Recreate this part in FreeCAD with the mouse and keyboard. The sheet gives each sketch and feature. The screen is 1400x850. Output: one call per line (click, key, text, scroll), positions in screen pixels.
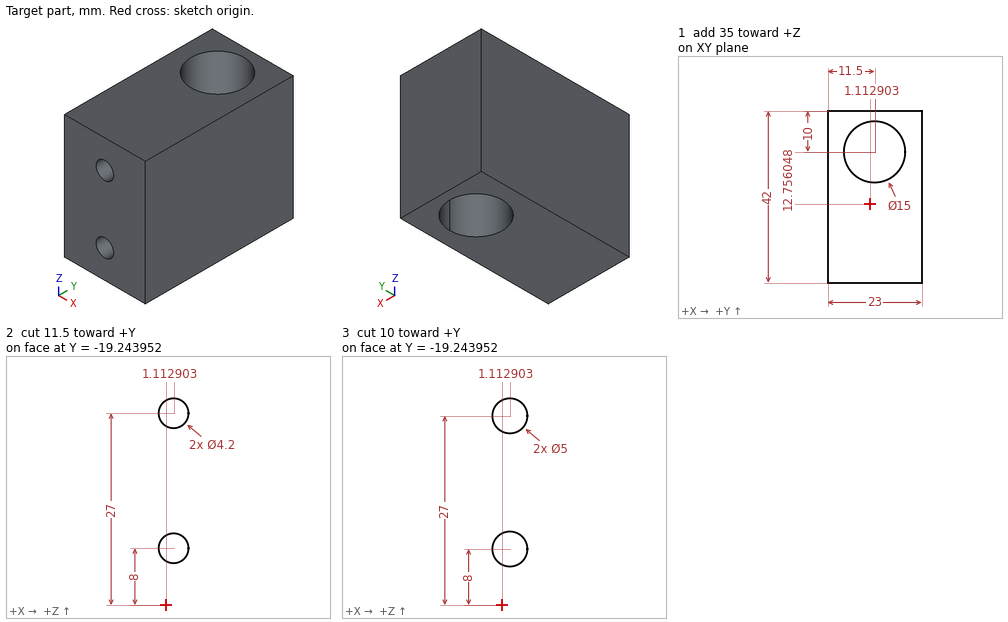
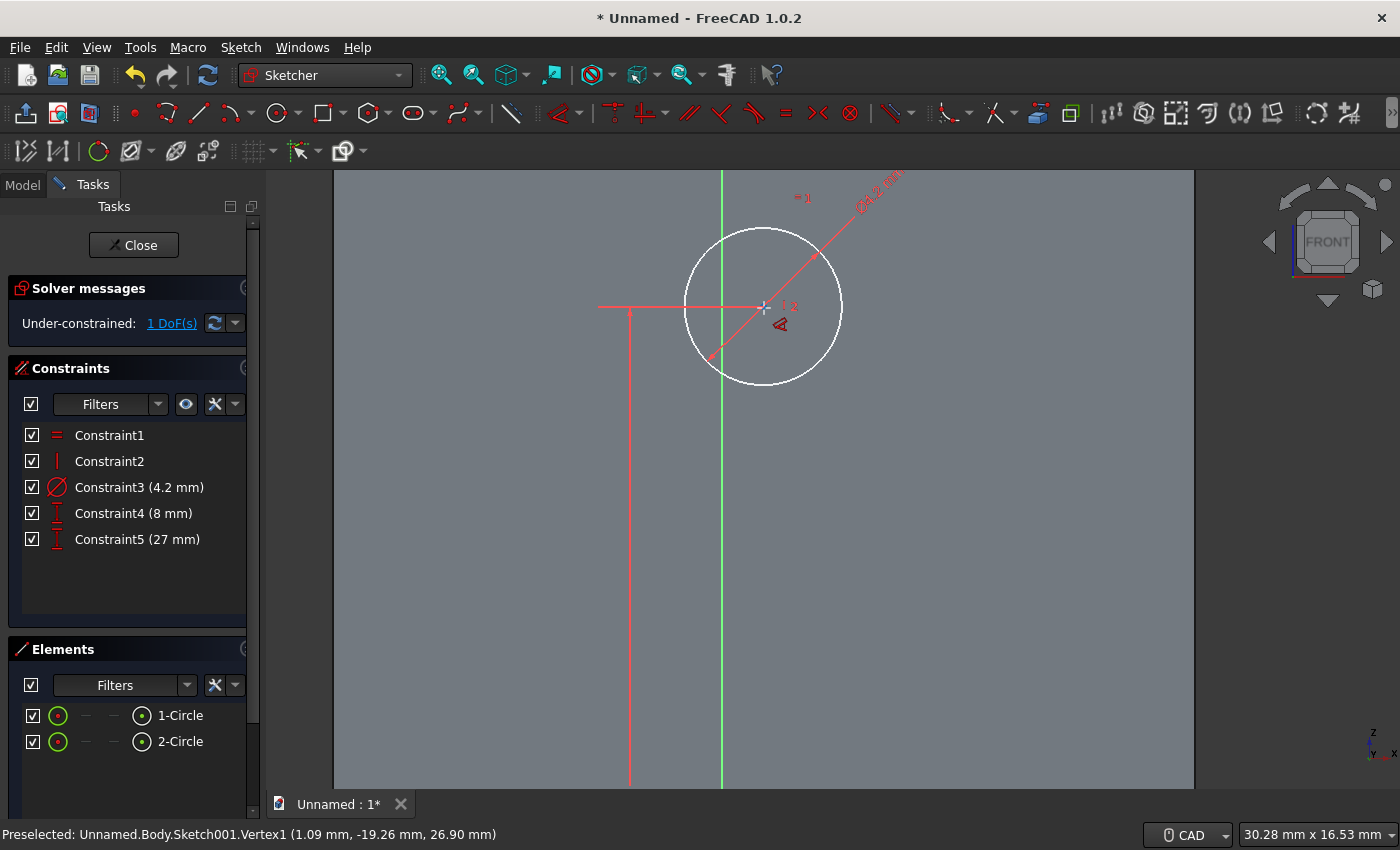
click(763, 307)
click(743, 273)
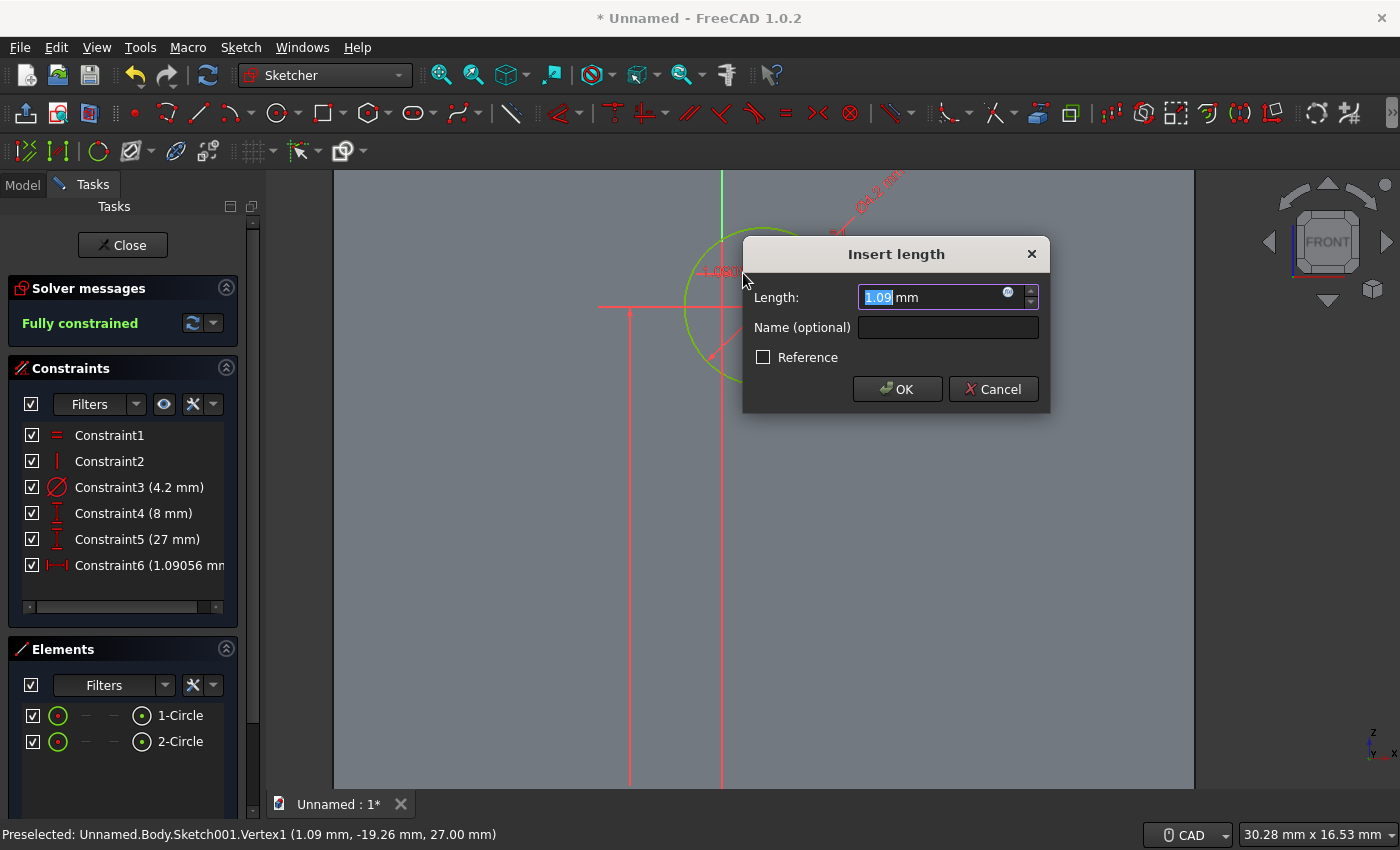
text(1.112903)
key(Return)
key(Escape)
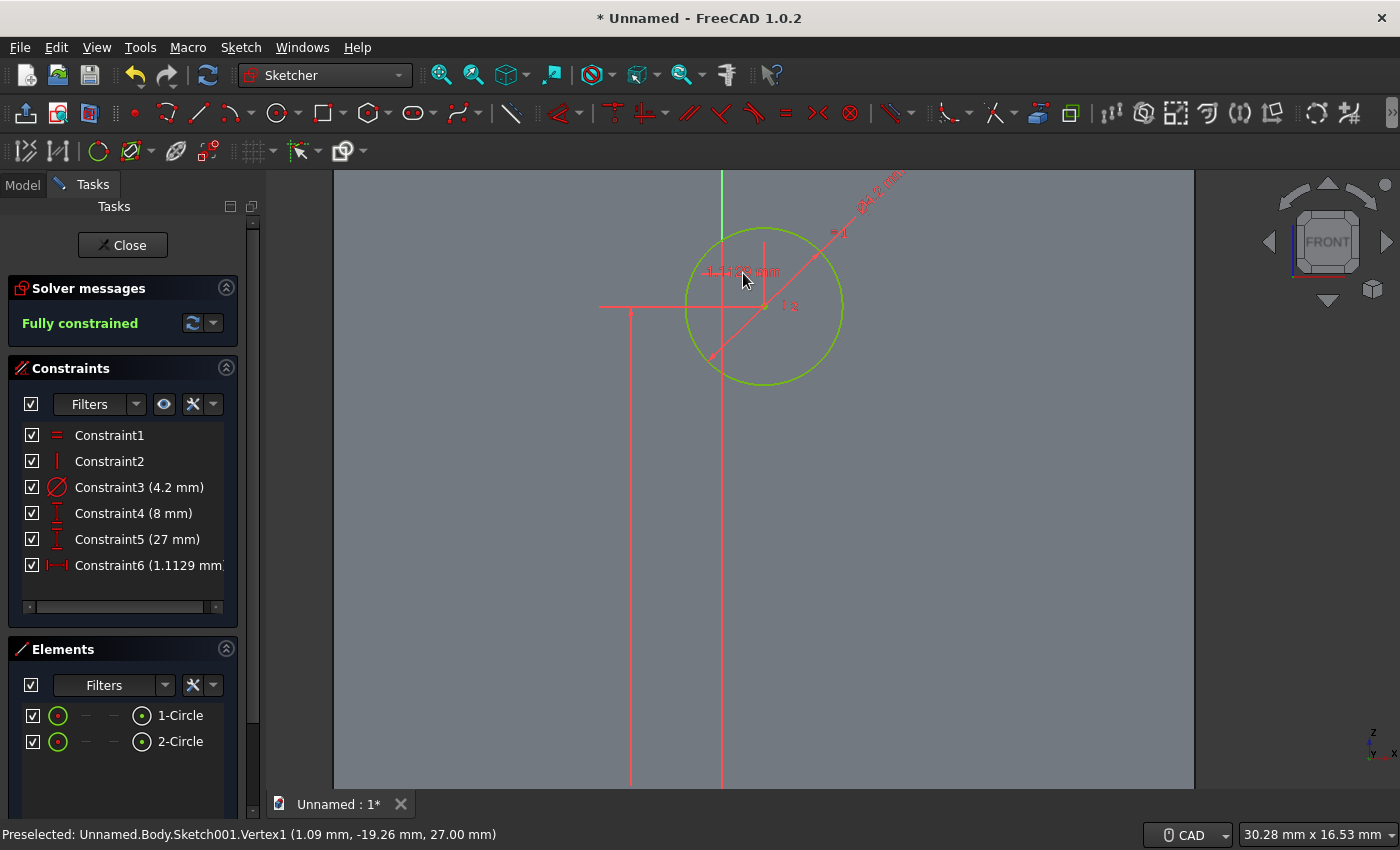
click(123, 245)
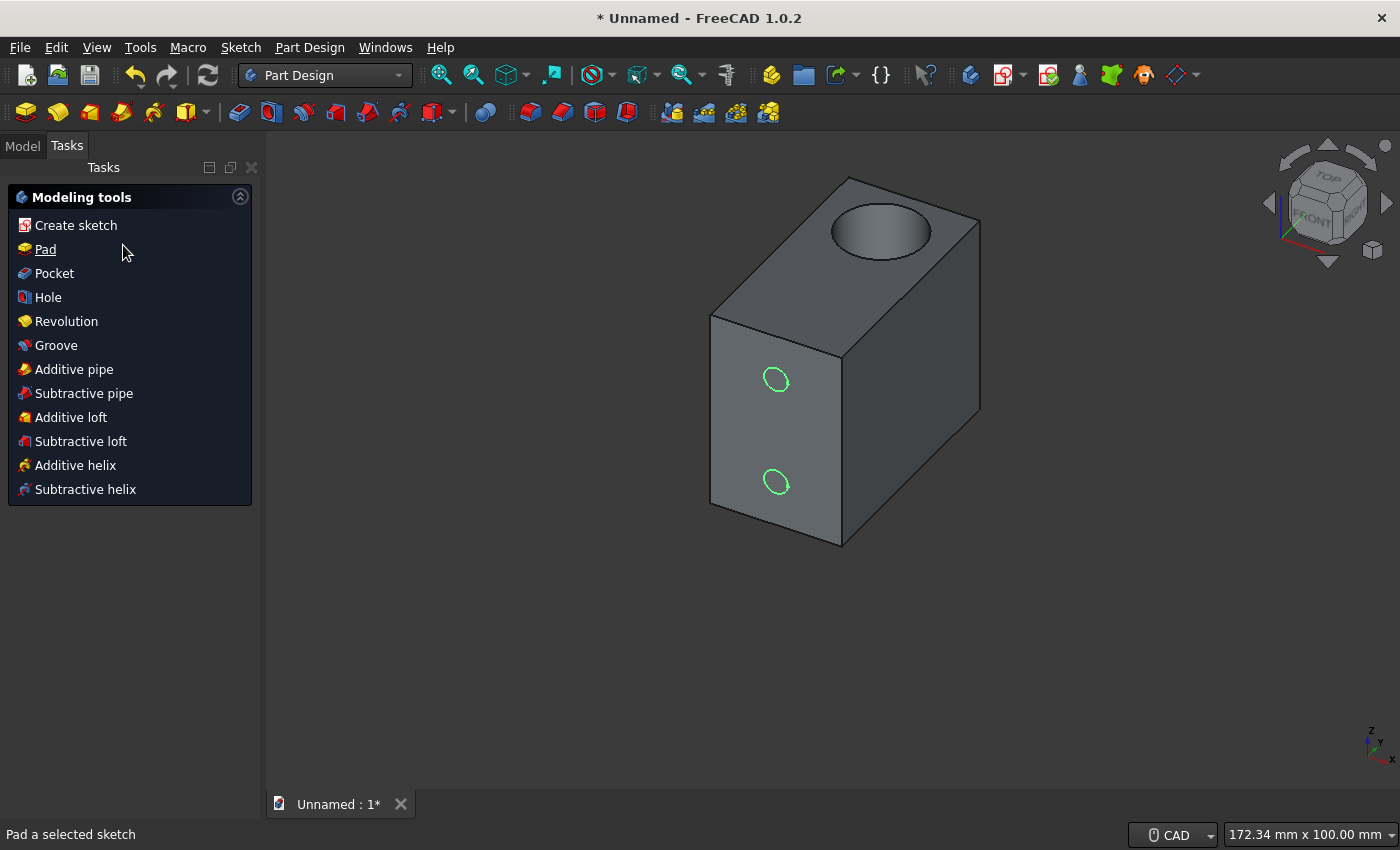
click(240, 112)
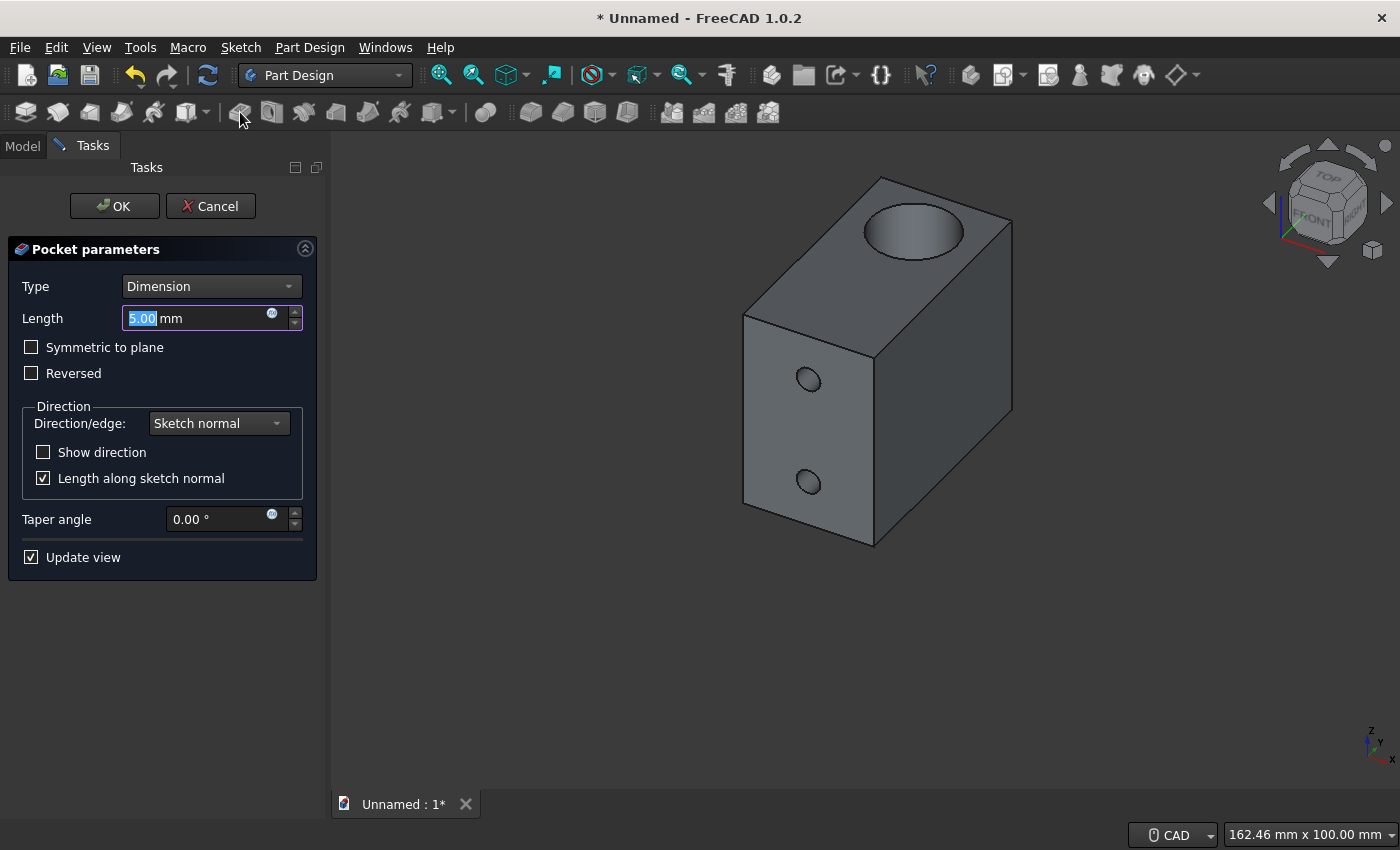
text(11.5)
key(Tab)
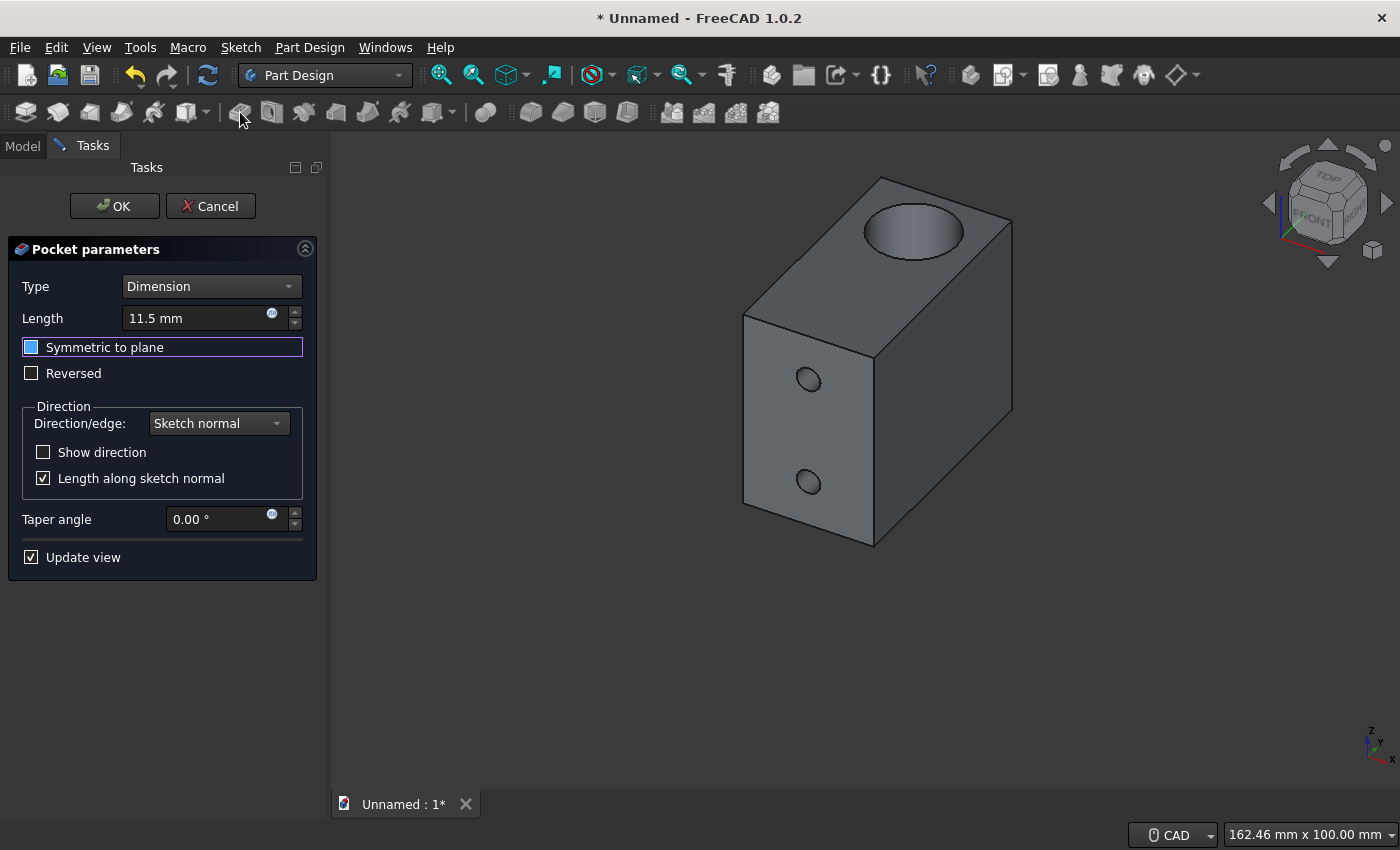
click(115, 206)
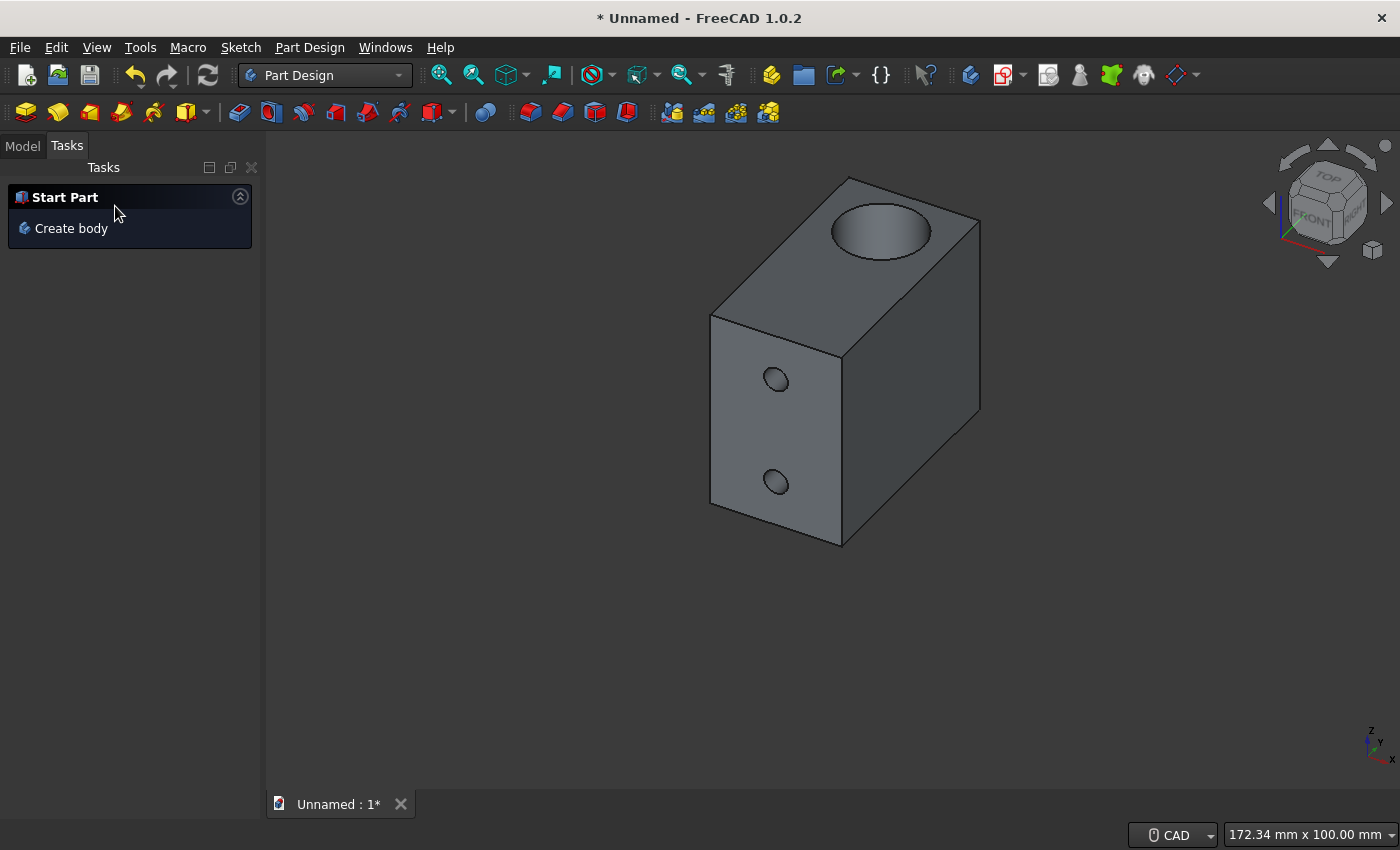
click(795, 436)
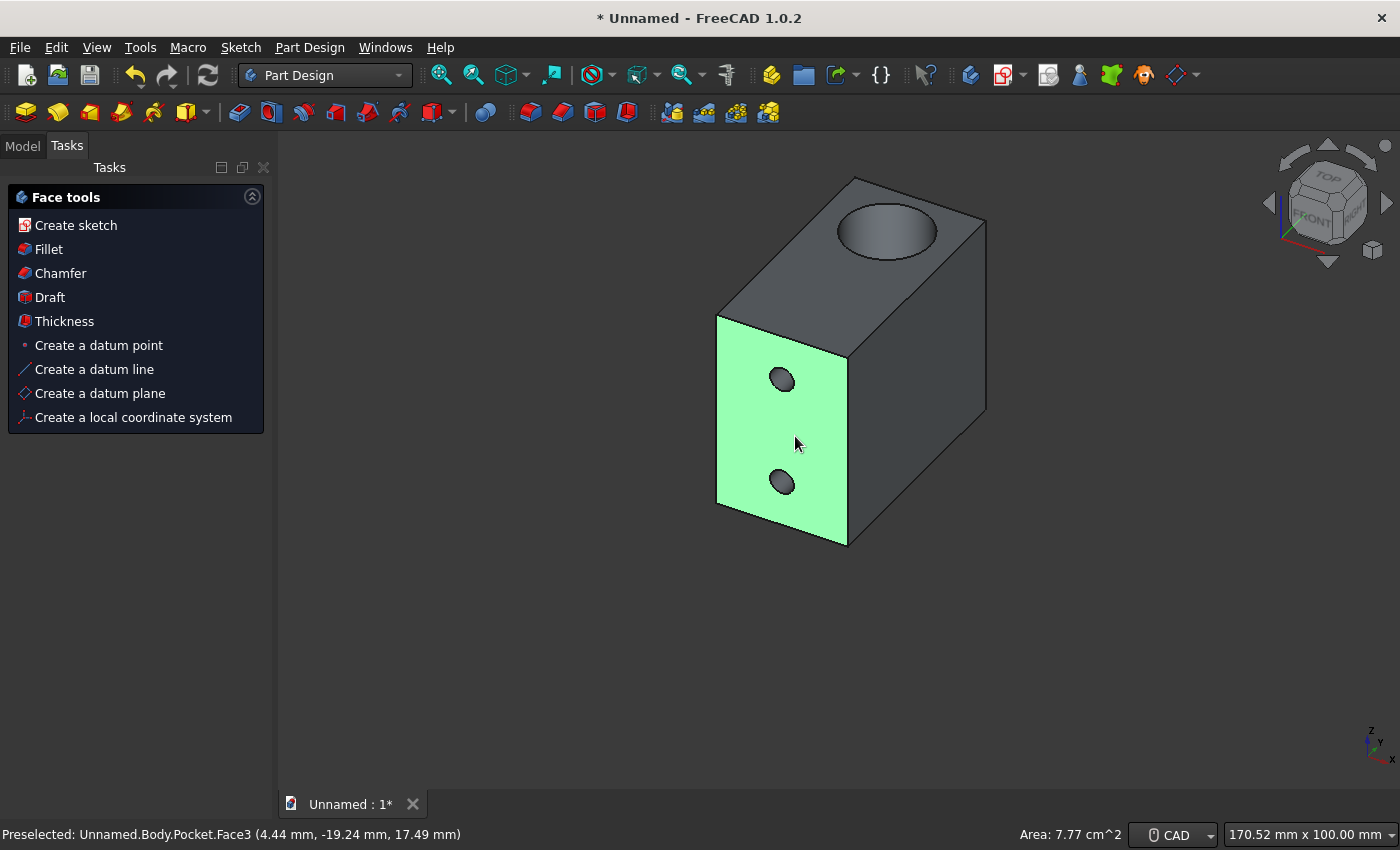
click(1004, 76)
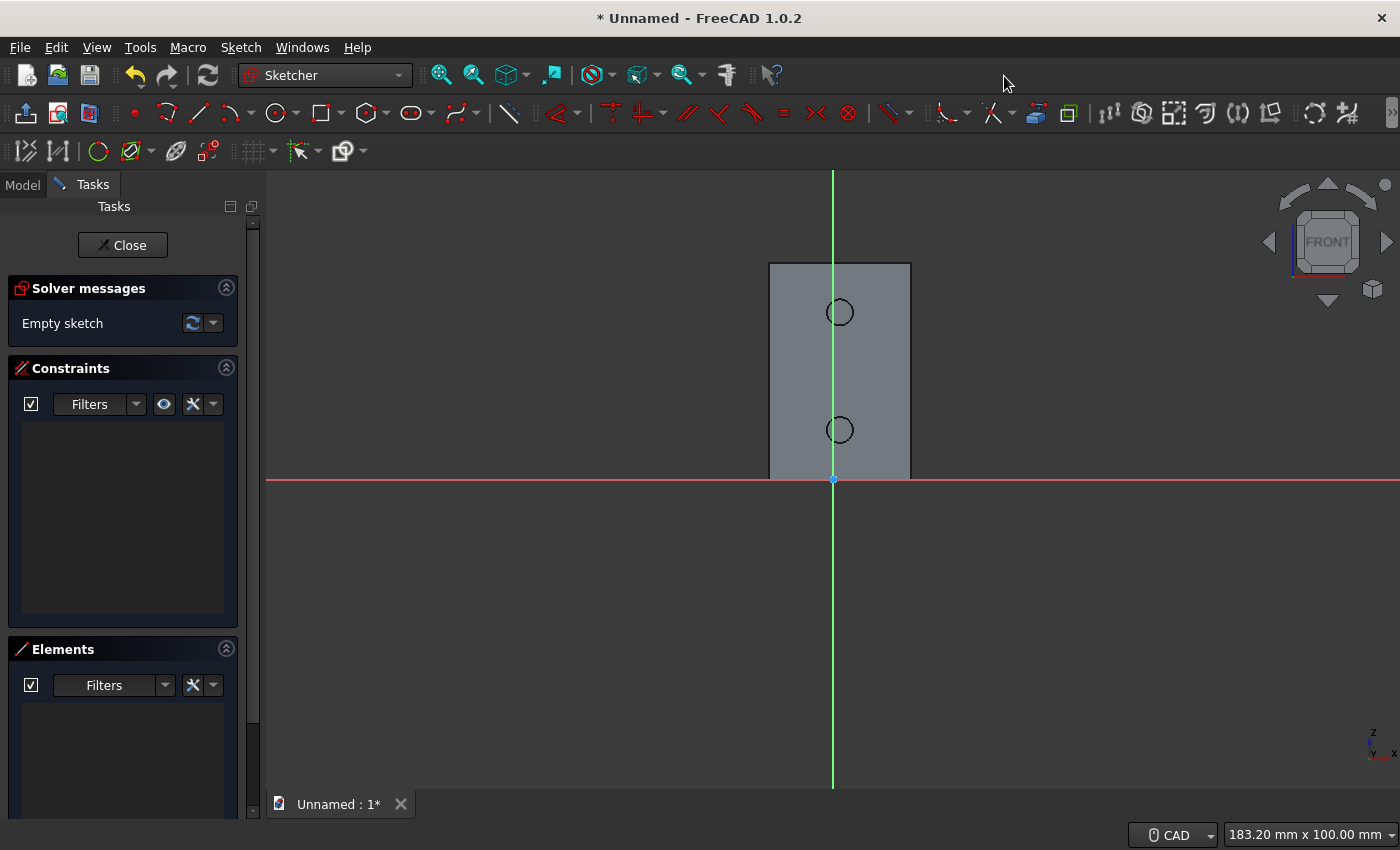
scroll(901, 314, up, 4)